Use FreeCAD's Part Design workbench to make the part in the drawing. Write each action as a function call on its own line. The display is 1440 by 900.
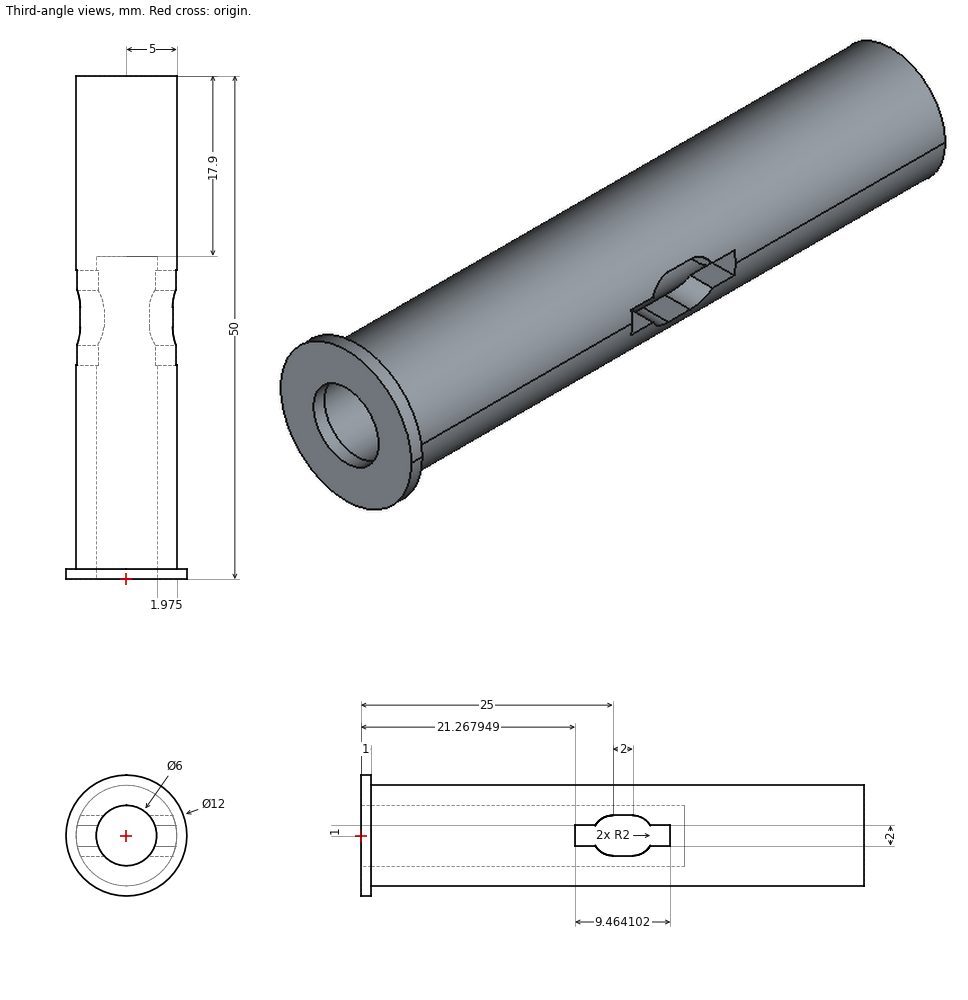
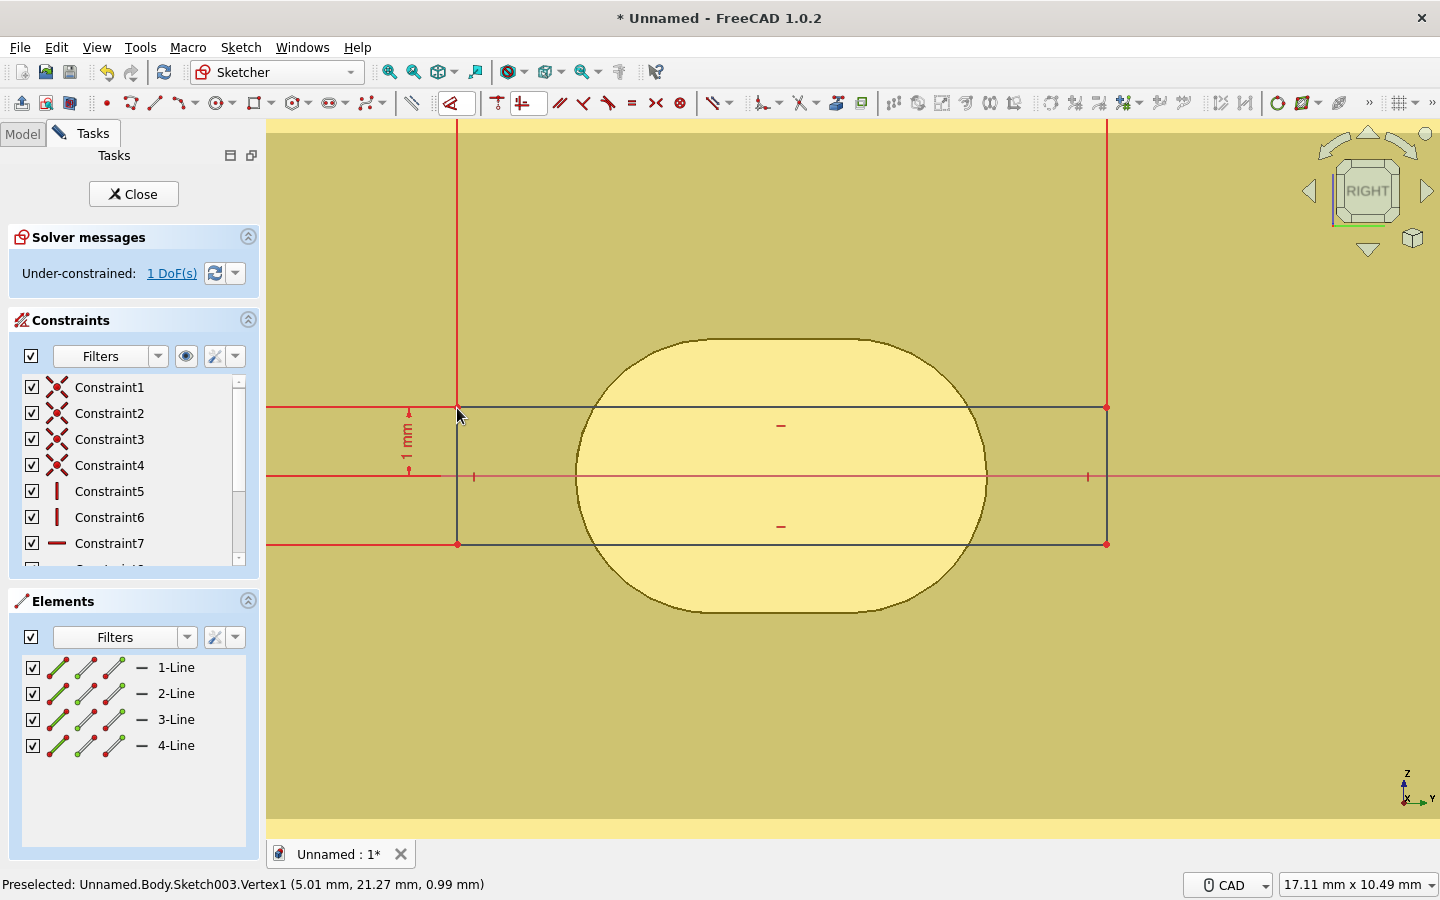
click(457, 407)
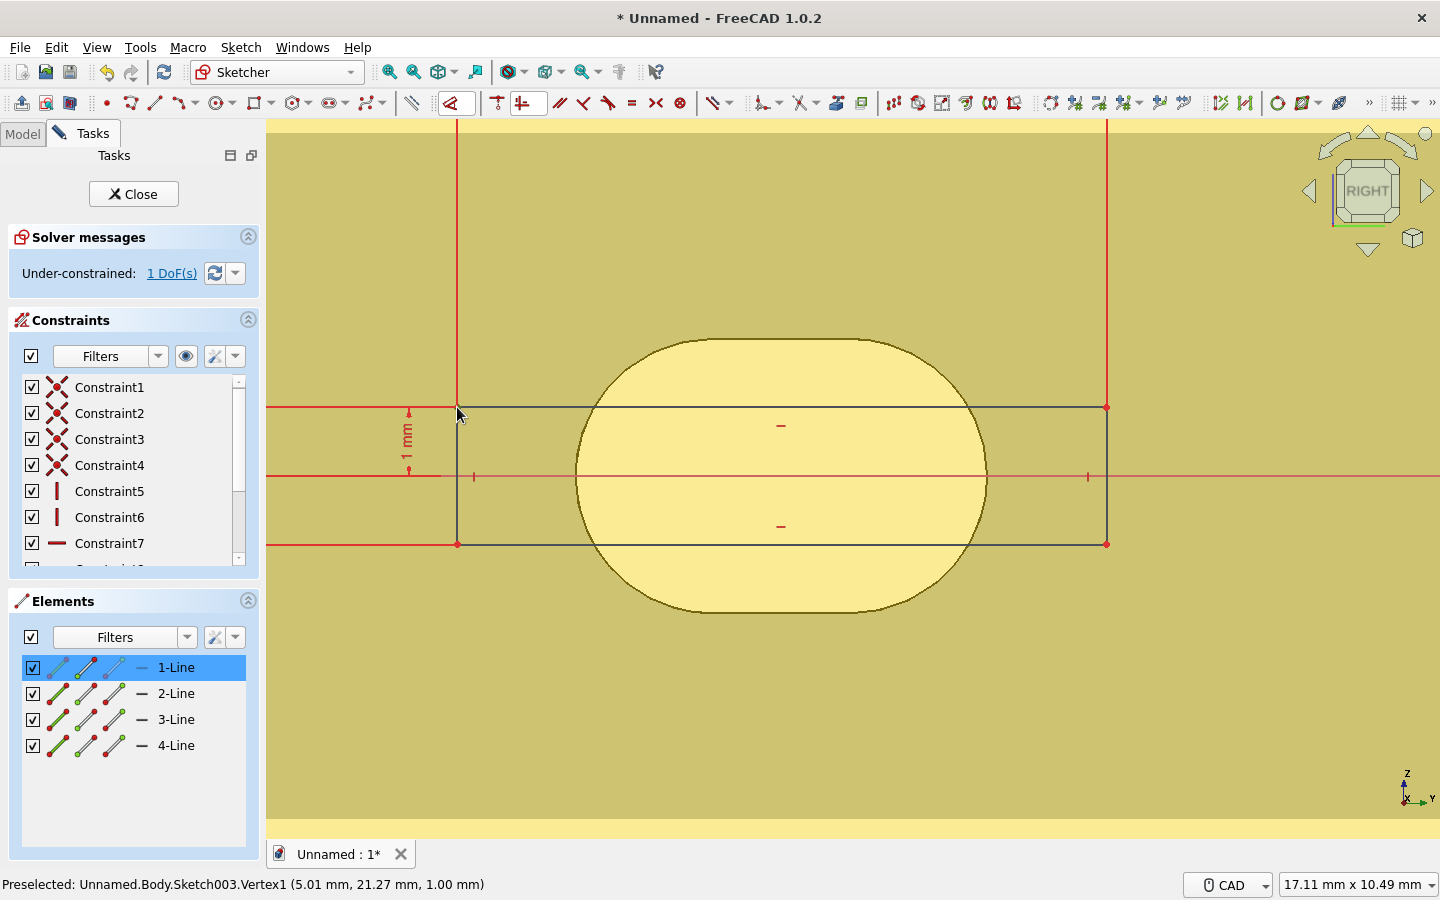
click(470, 104)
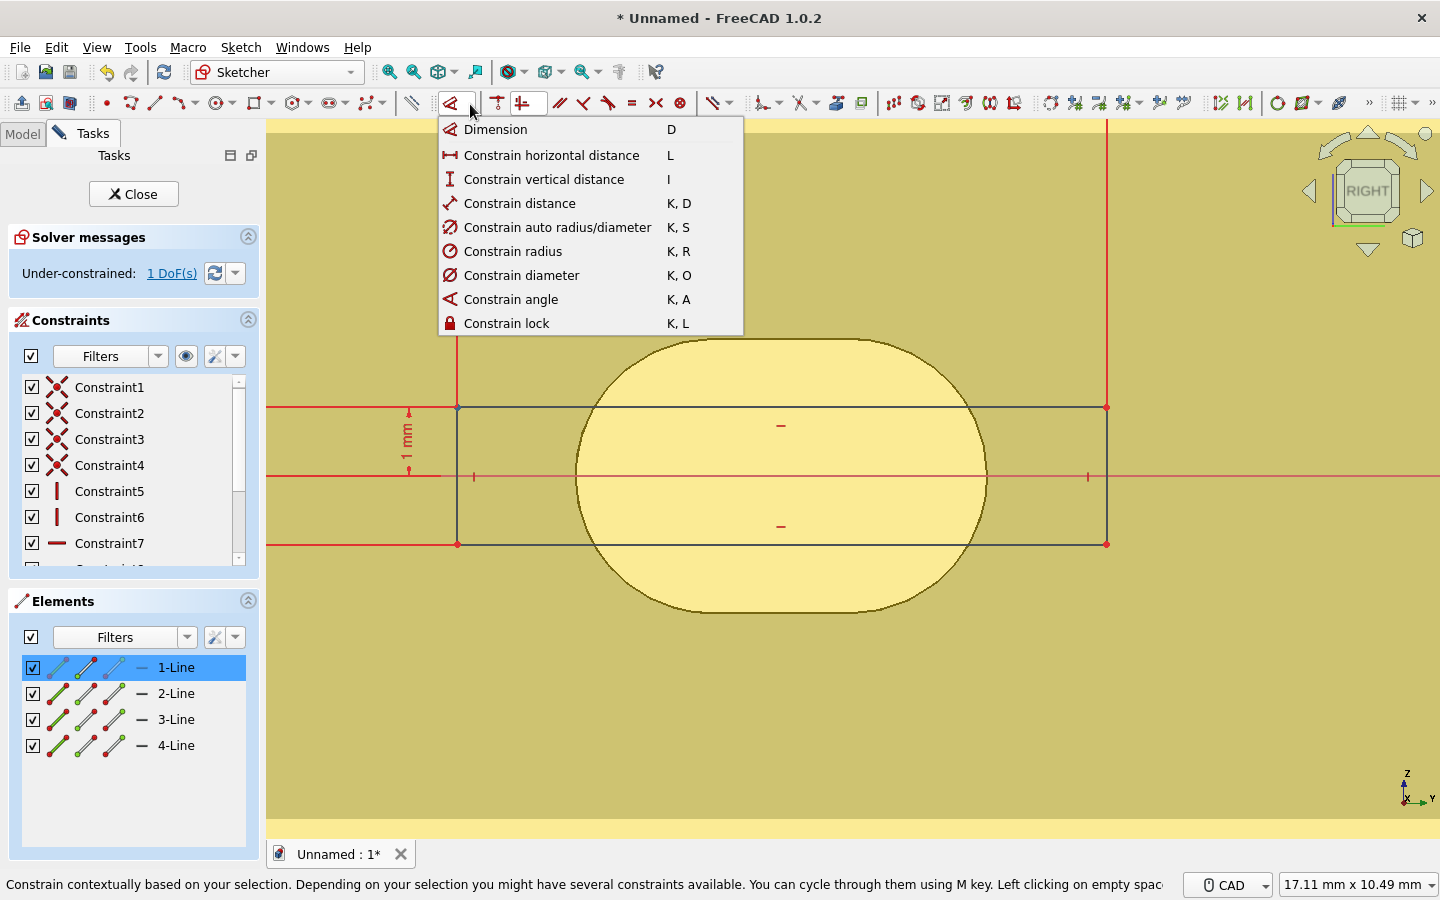
click(591, 155)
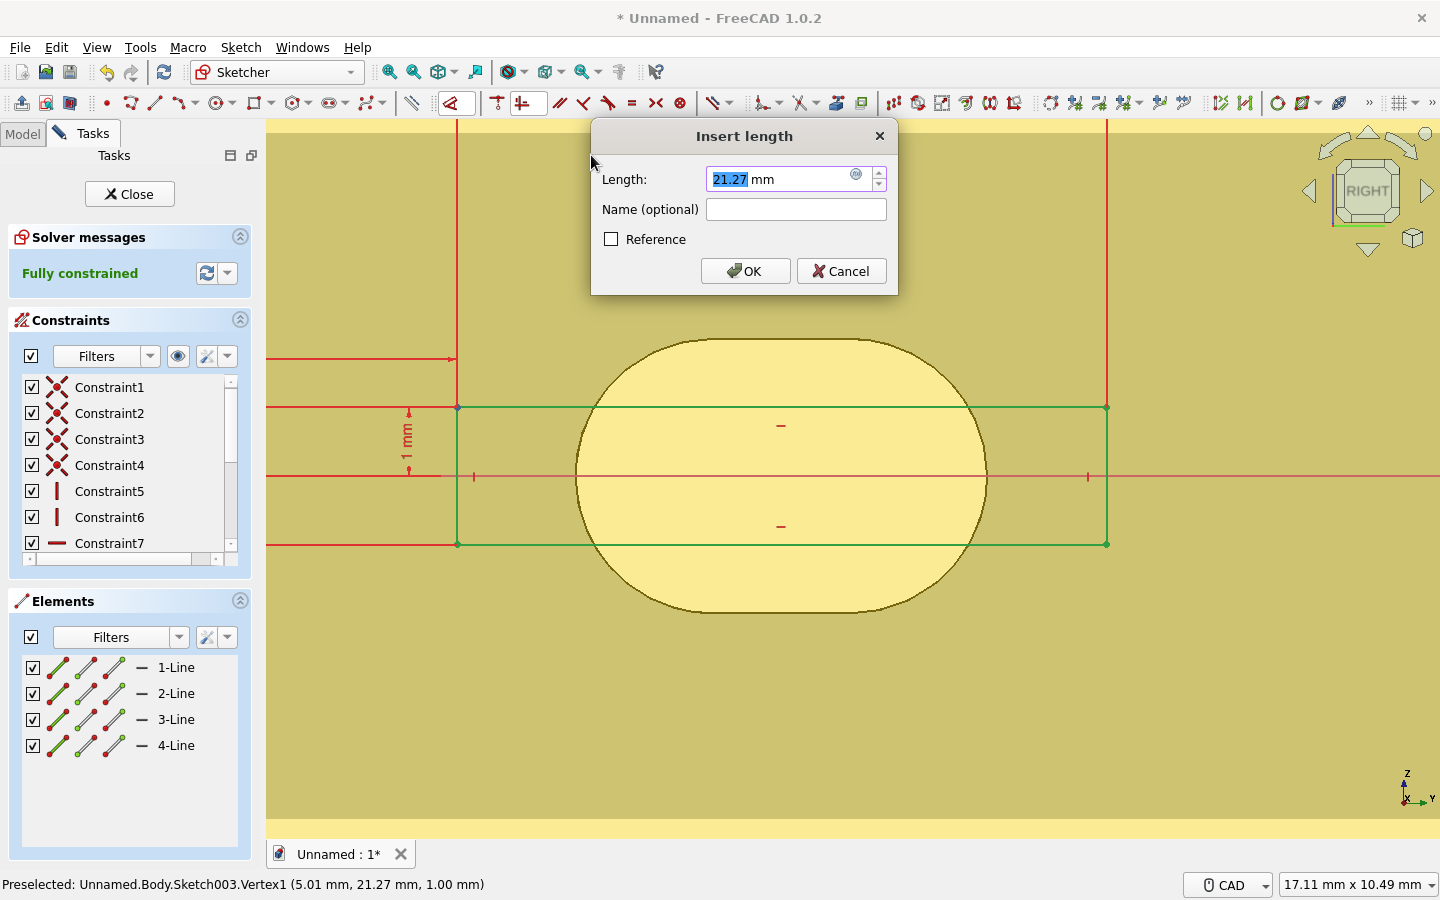
text(21.267949)
key(Return)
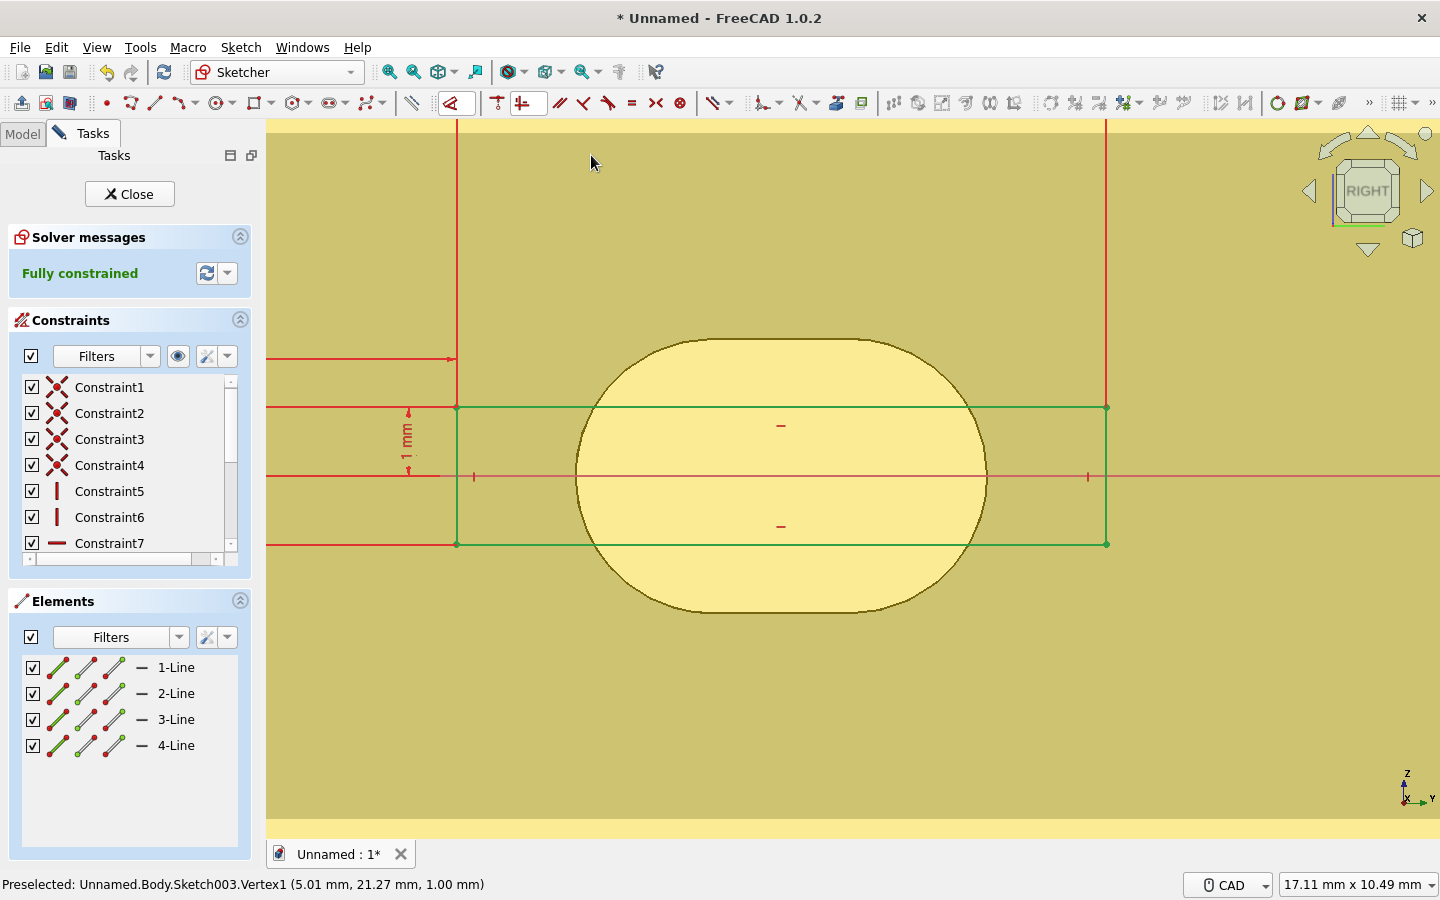
click(130, 194)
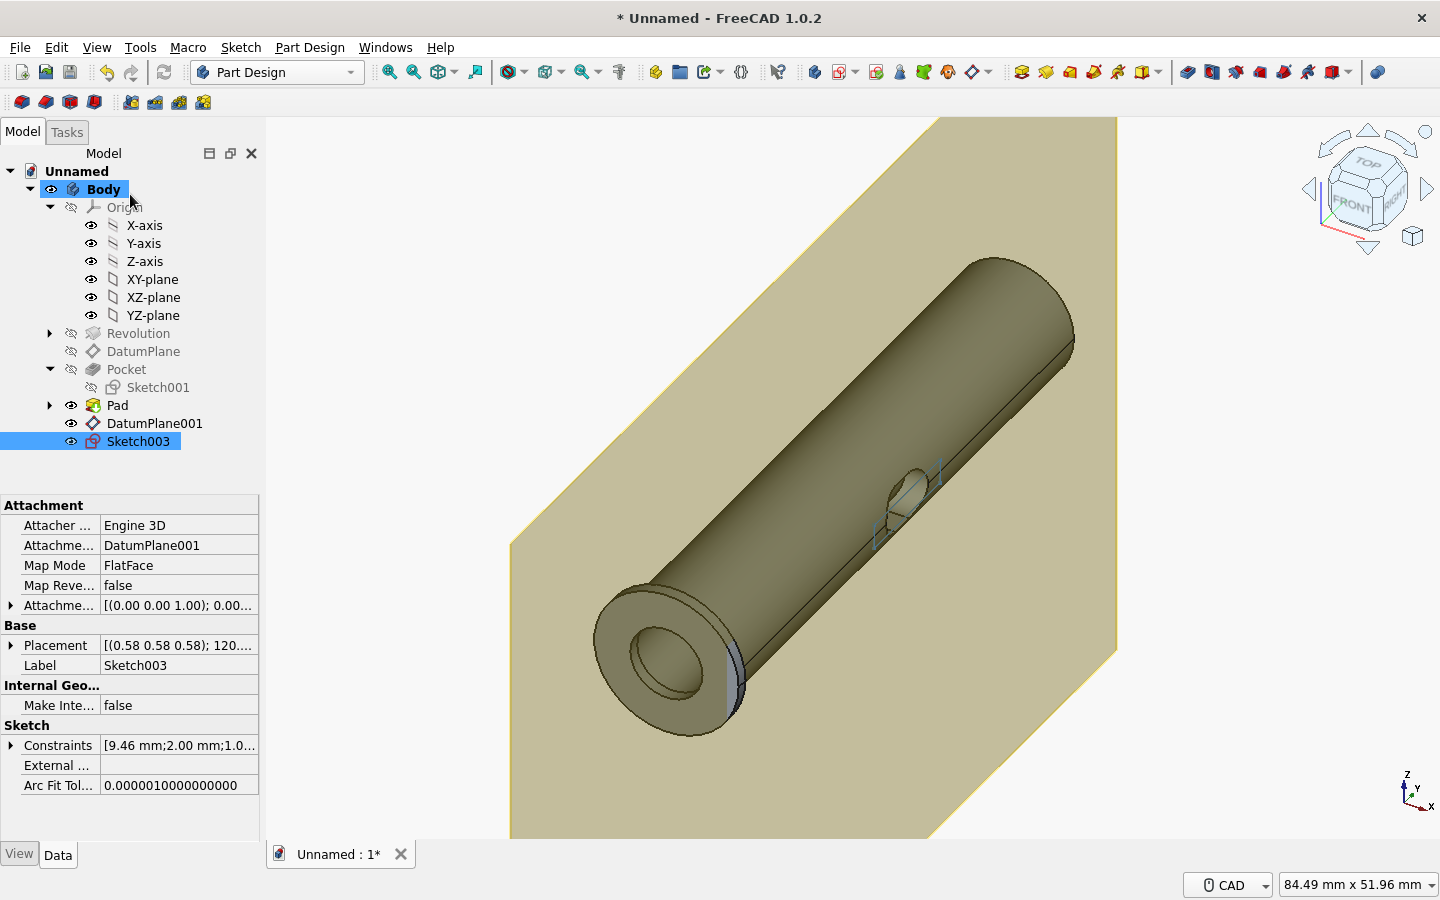
click(1188, 72)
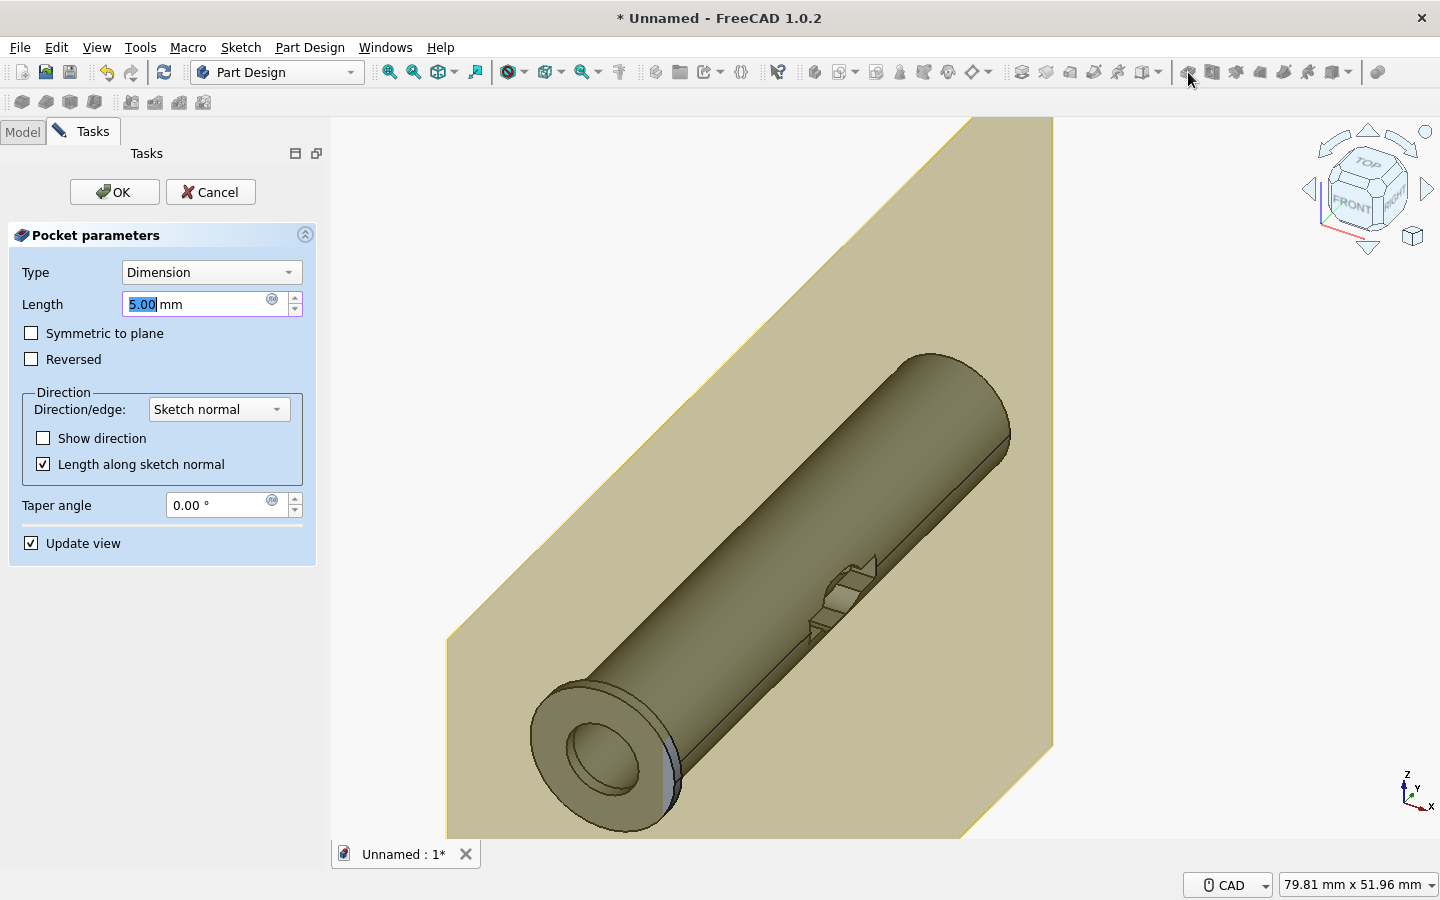
click(212, 272)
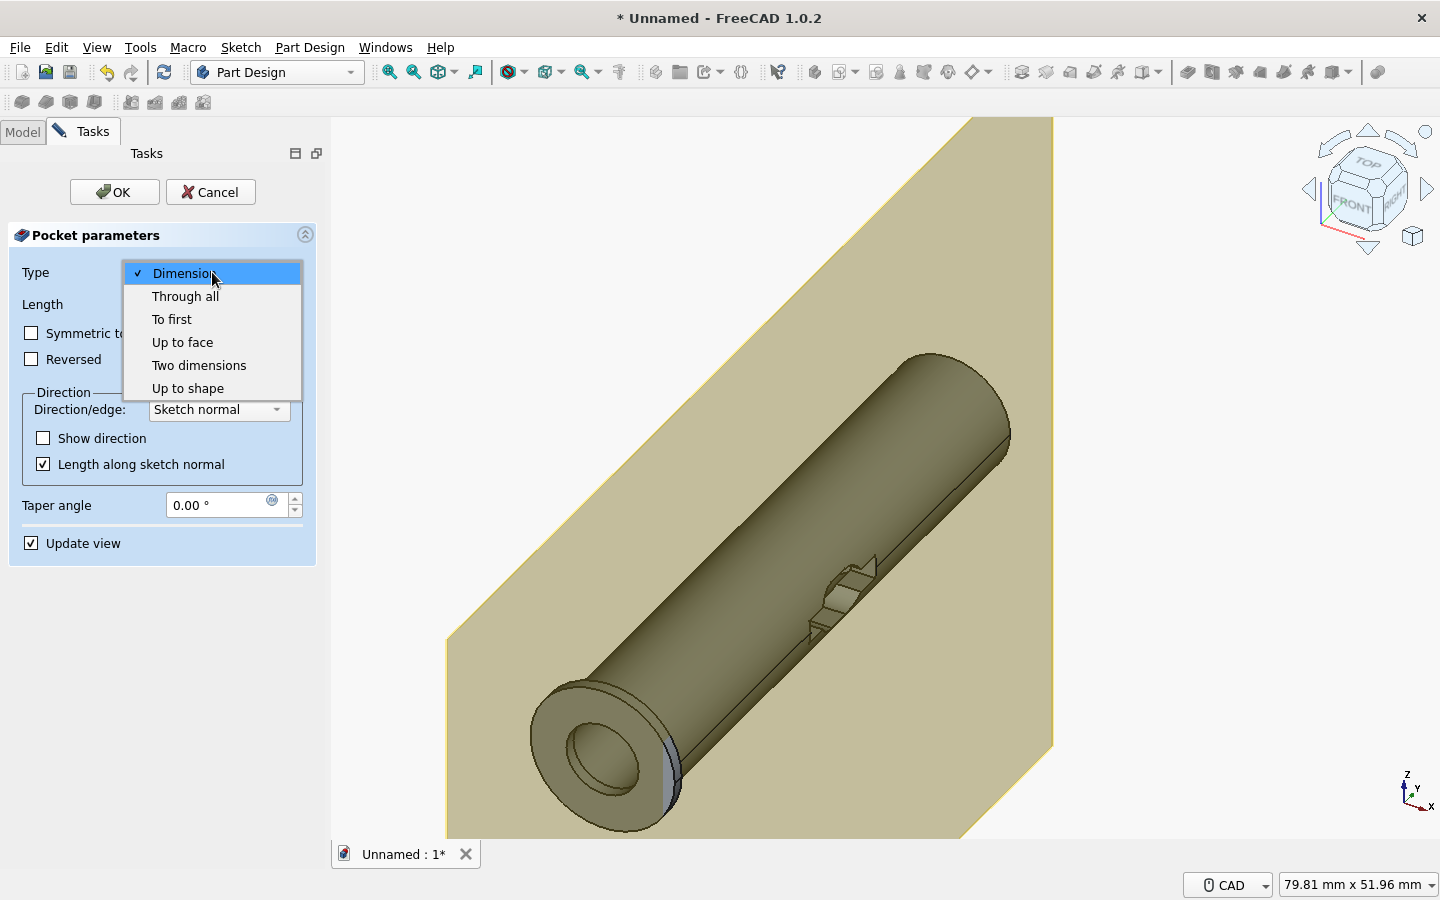
click(212, 296)